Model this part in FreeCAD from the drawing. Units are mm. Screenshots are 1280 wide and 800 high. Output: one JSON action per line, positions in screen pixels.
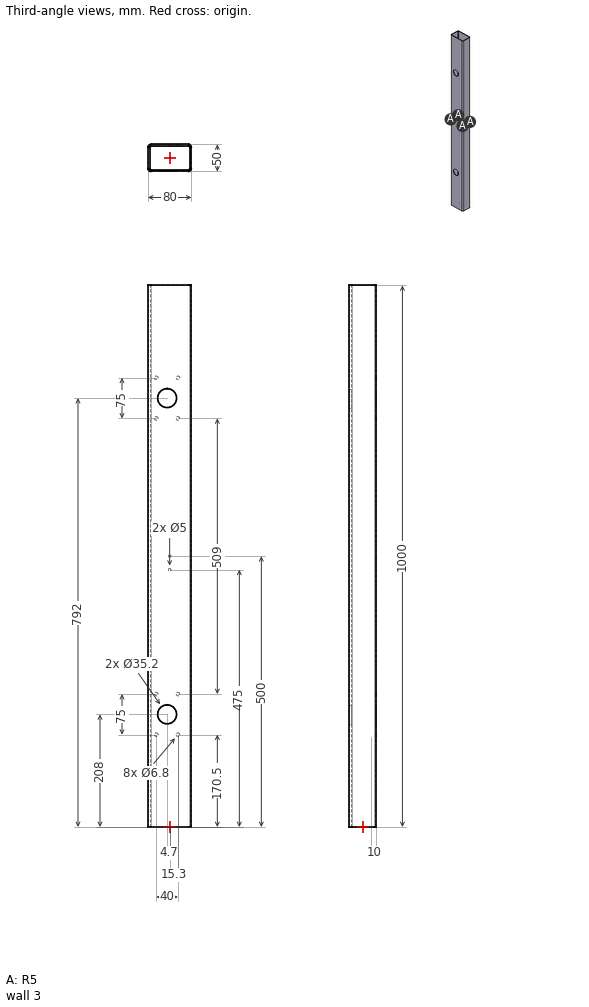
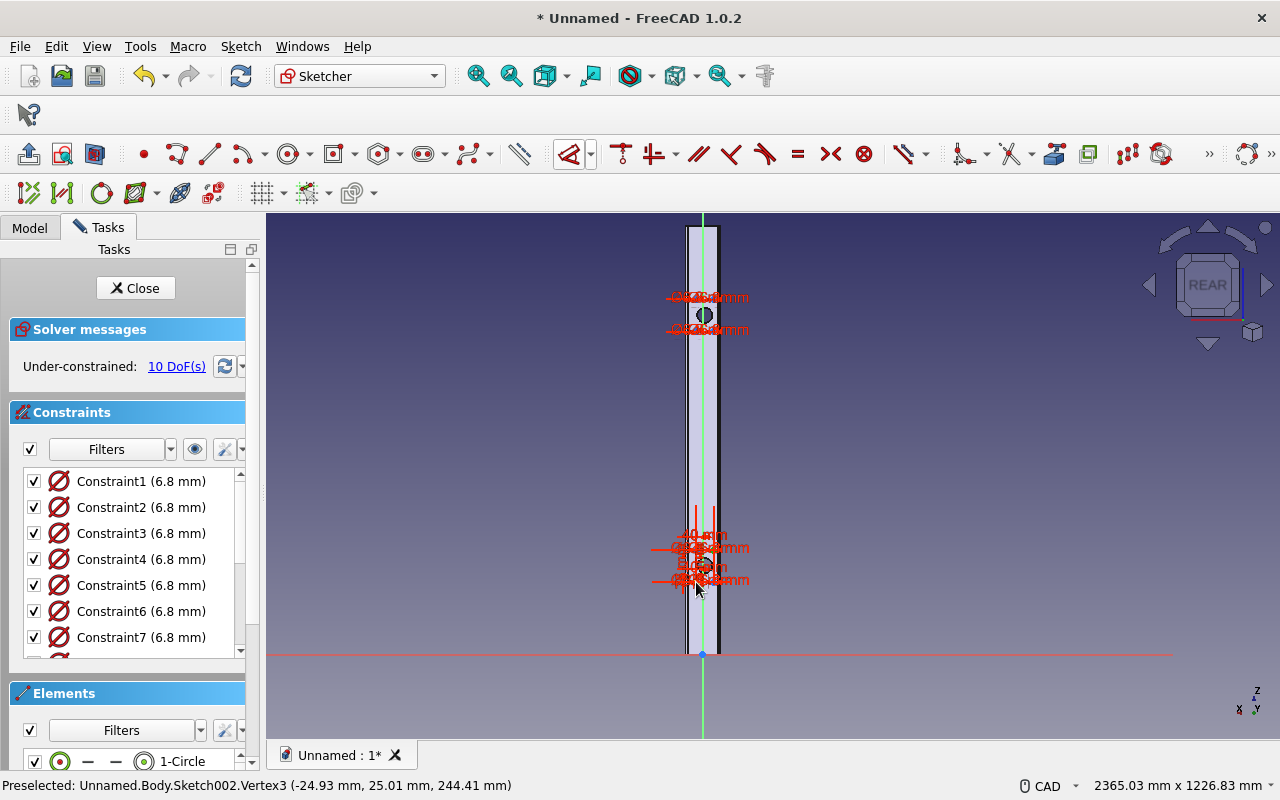
{"action": "scroll", "coordinate": [696, 332], "scroll_direction": "up", "scroll_amount": 5}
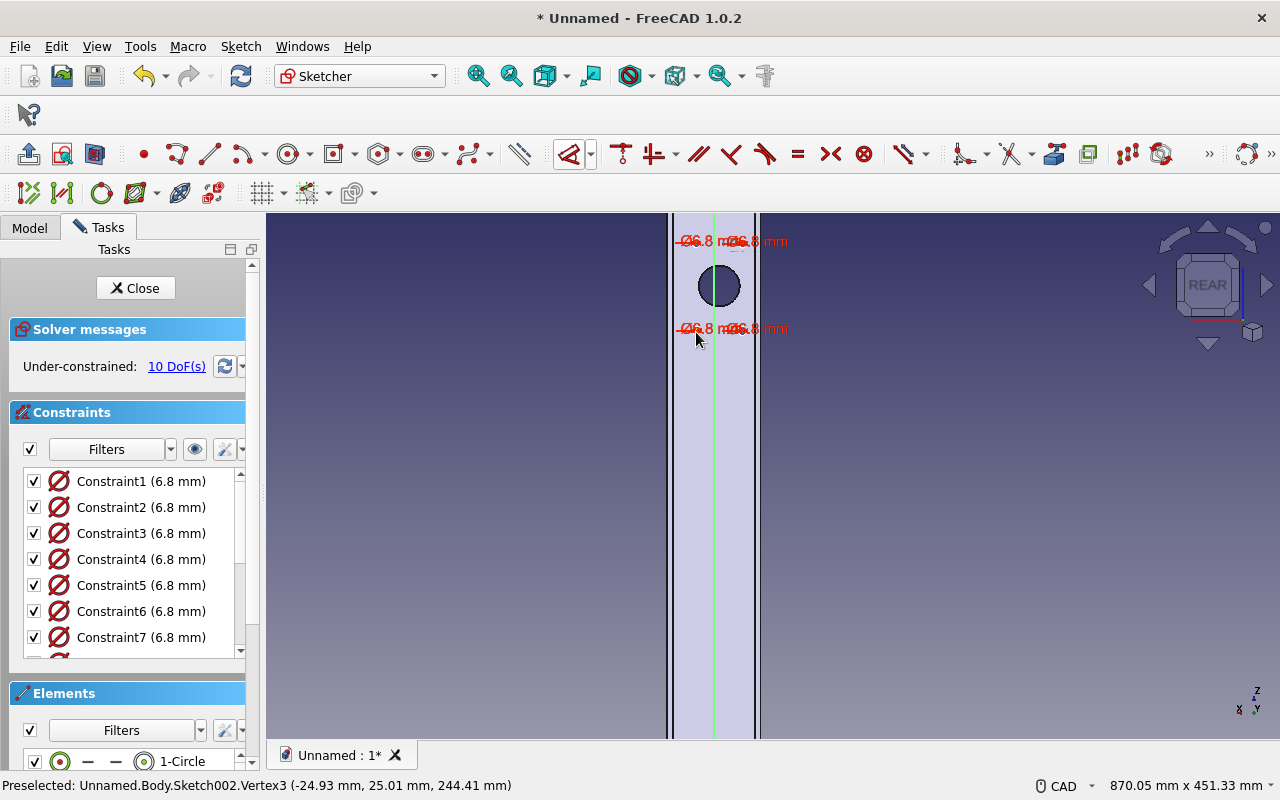
{"action": "left_click", "coordinate": [696, 331]}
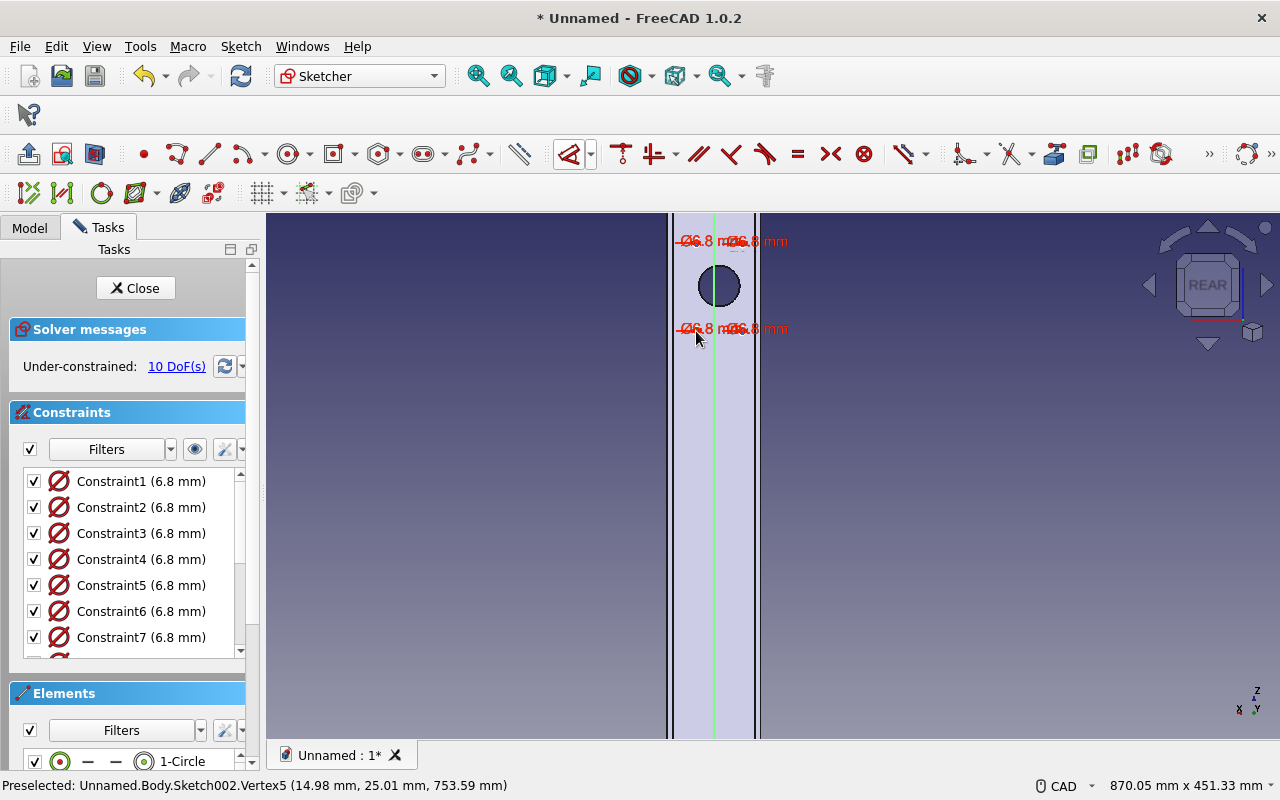
{"action": "key", "text": "l"}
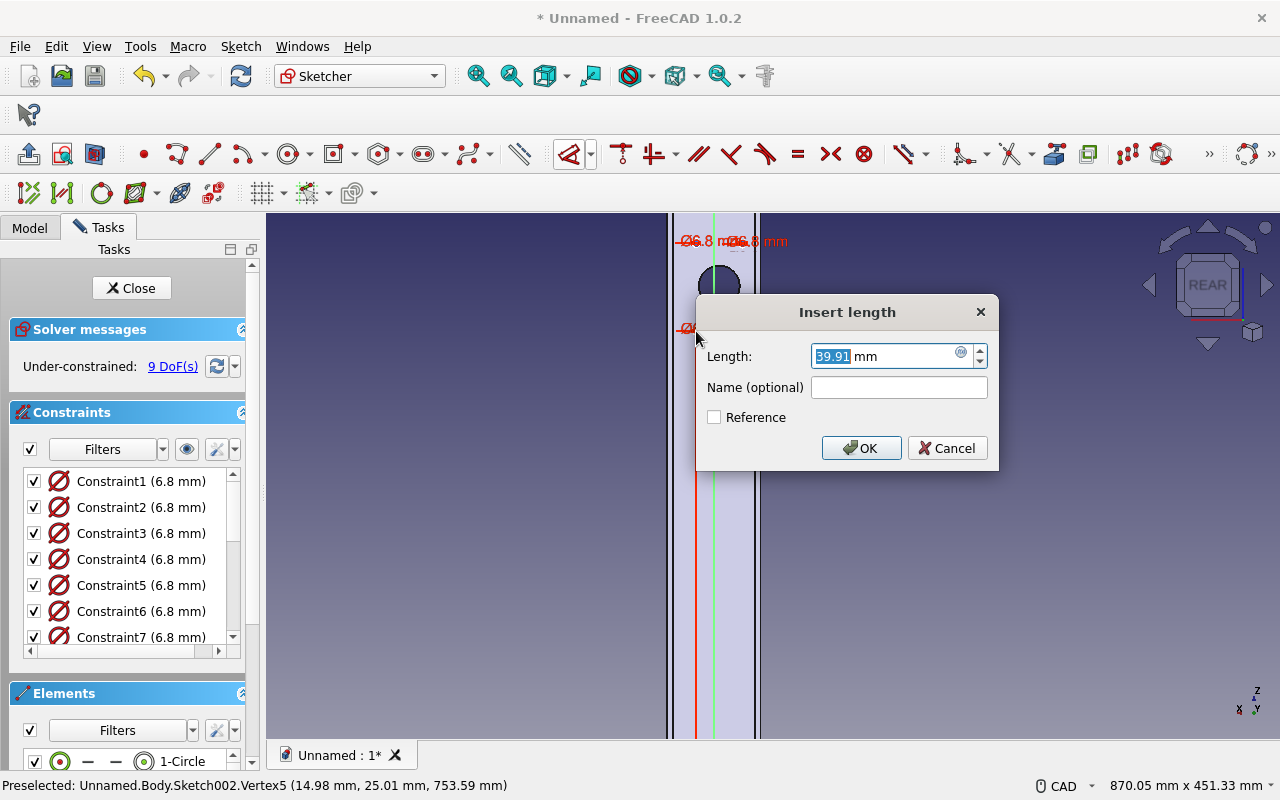
{"action": "type", "text": "40"}
{"action": "key", "text": "Return"}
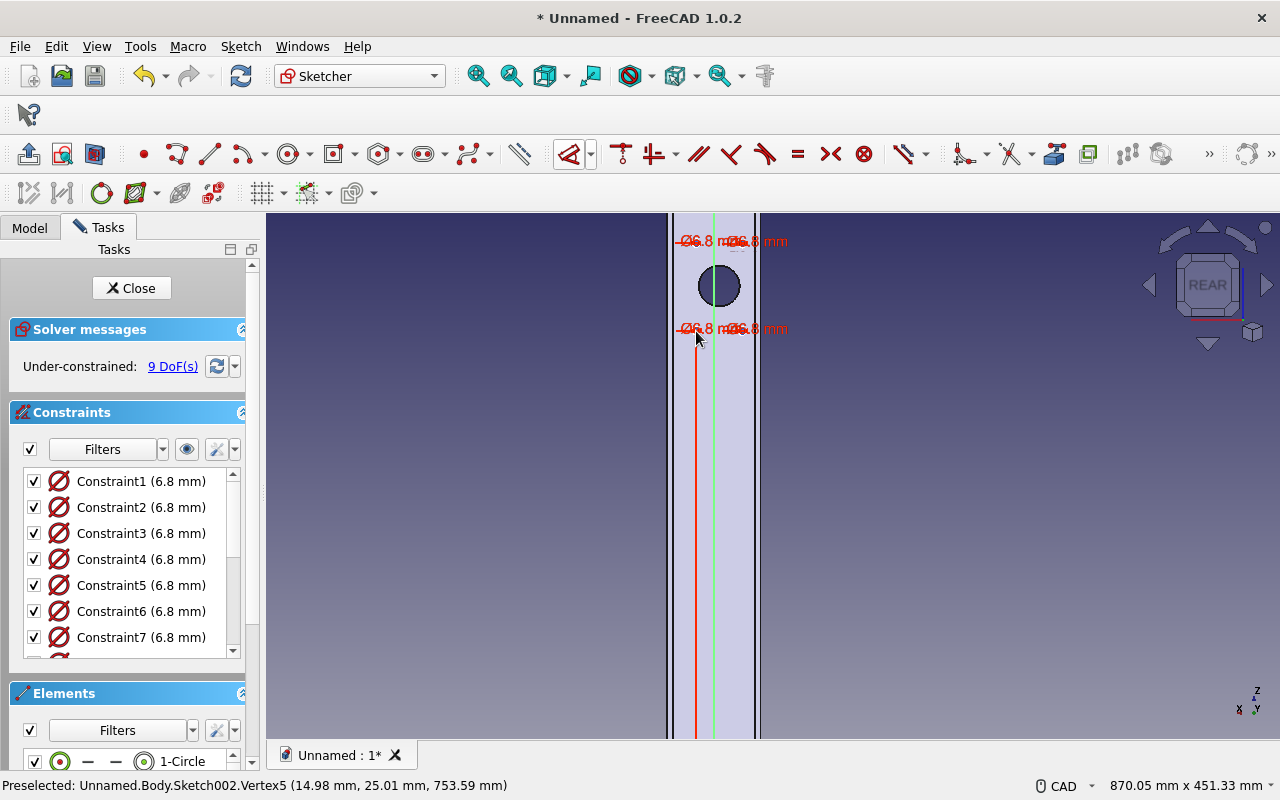
{"action": "left_click", "coordinate": [696, 331]}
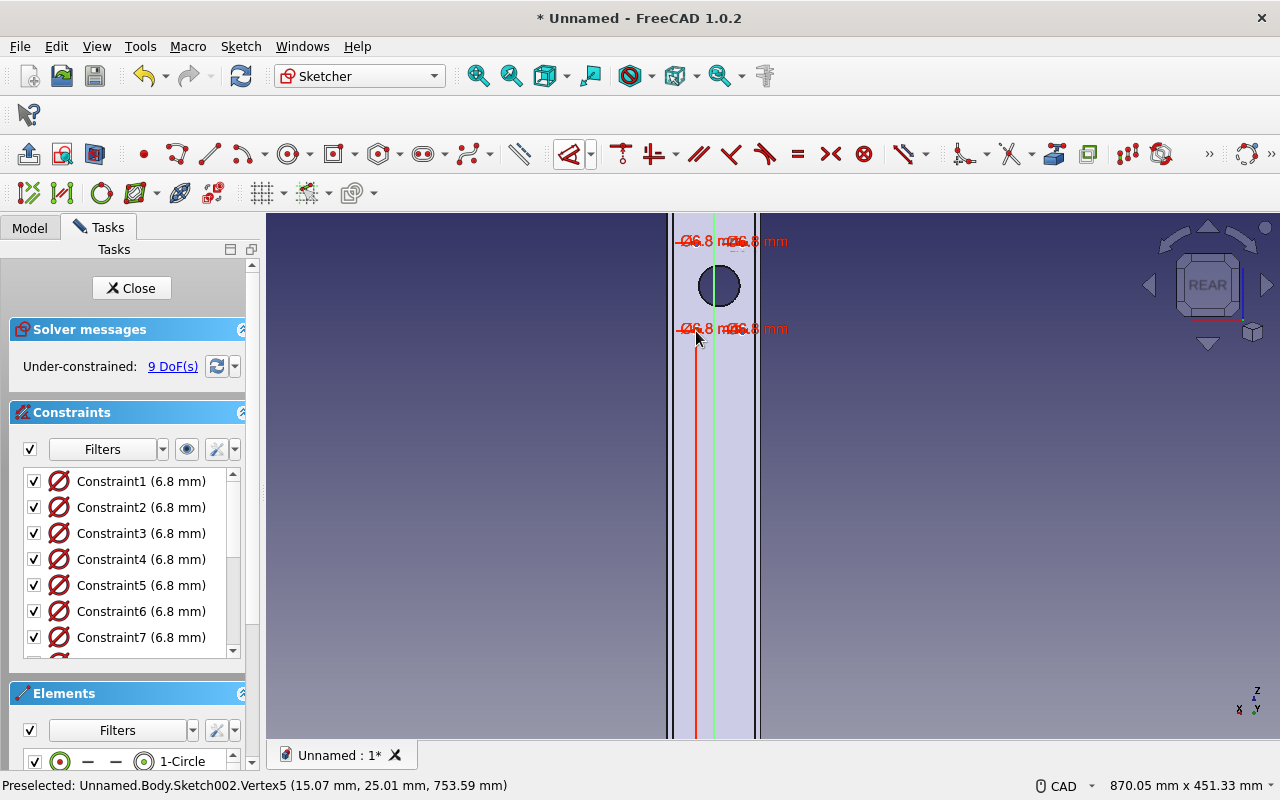
{"action": "left_click", "coordinate": [742, 331]}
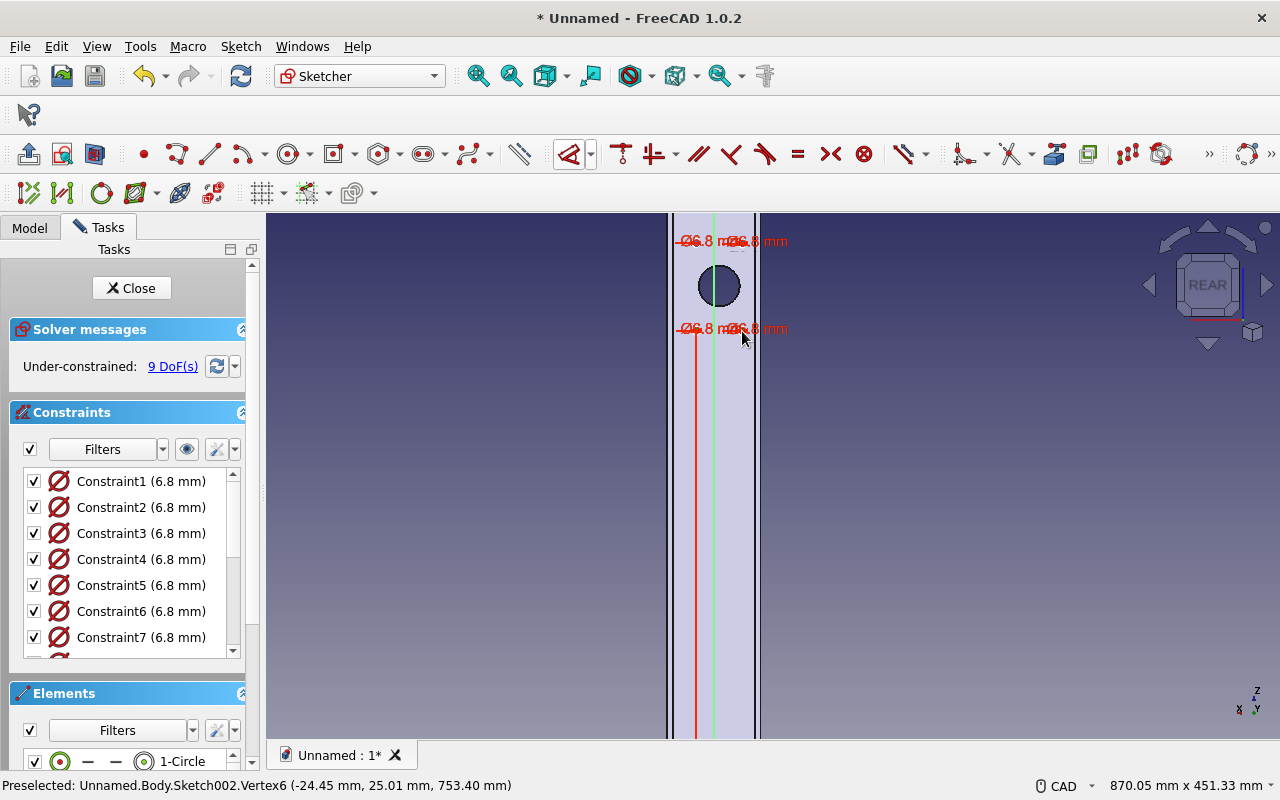
{"action": "left_click", "coordinate": [590, 154]}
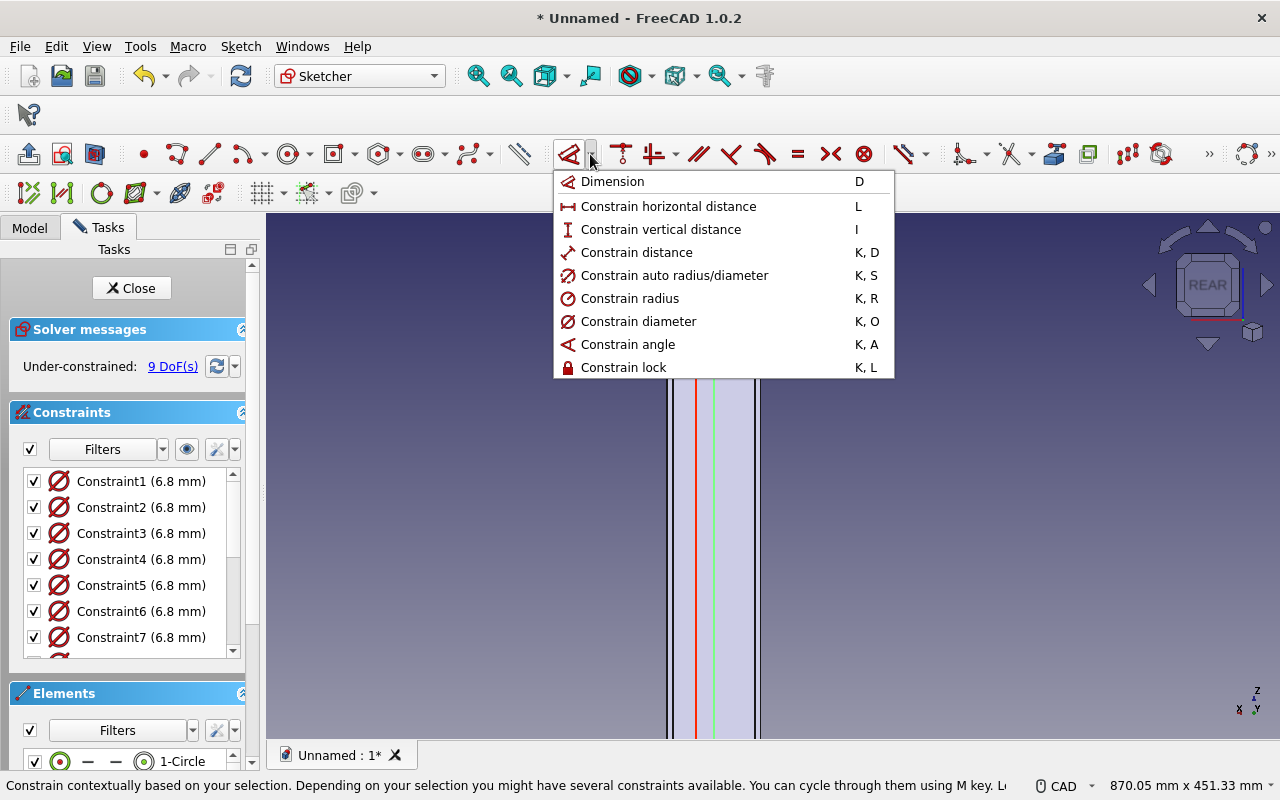
{"action": "left_click", "coordinate": [724, 206]}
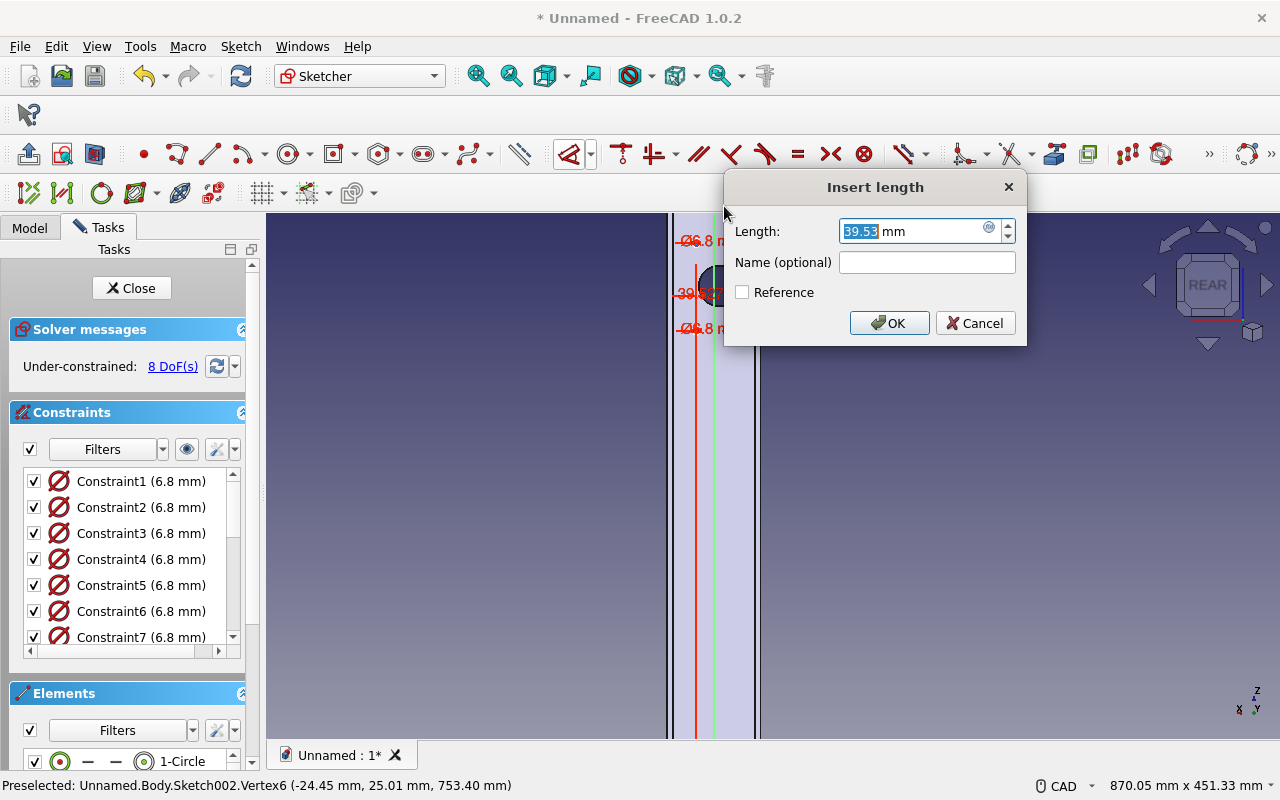
{"action": "type", "text": "40"}
{"action": "key", "text": "Return"}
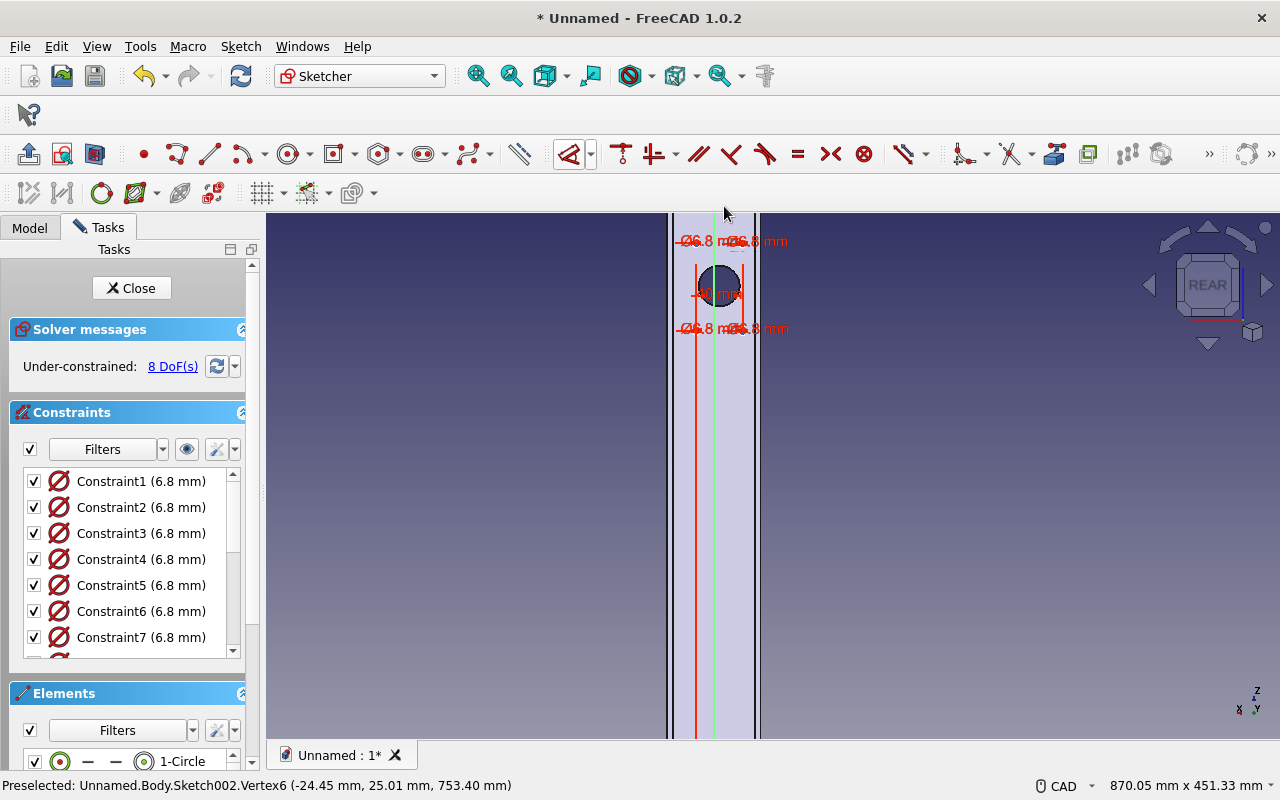
{"action": "left_click", "coordinate": [696, 331]}